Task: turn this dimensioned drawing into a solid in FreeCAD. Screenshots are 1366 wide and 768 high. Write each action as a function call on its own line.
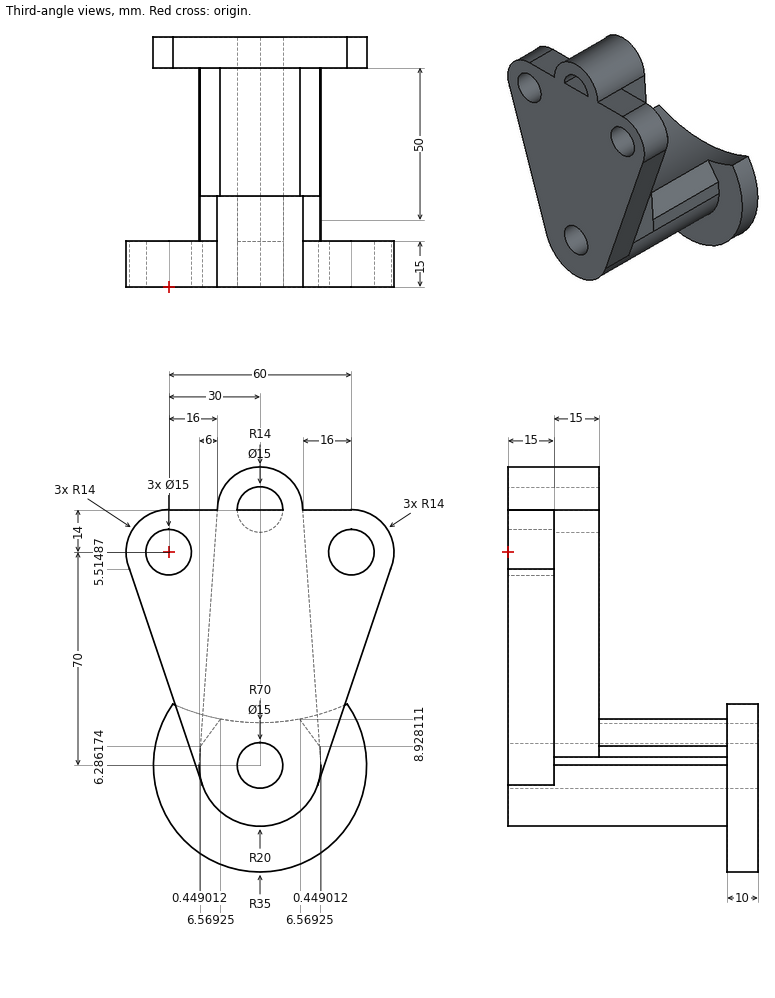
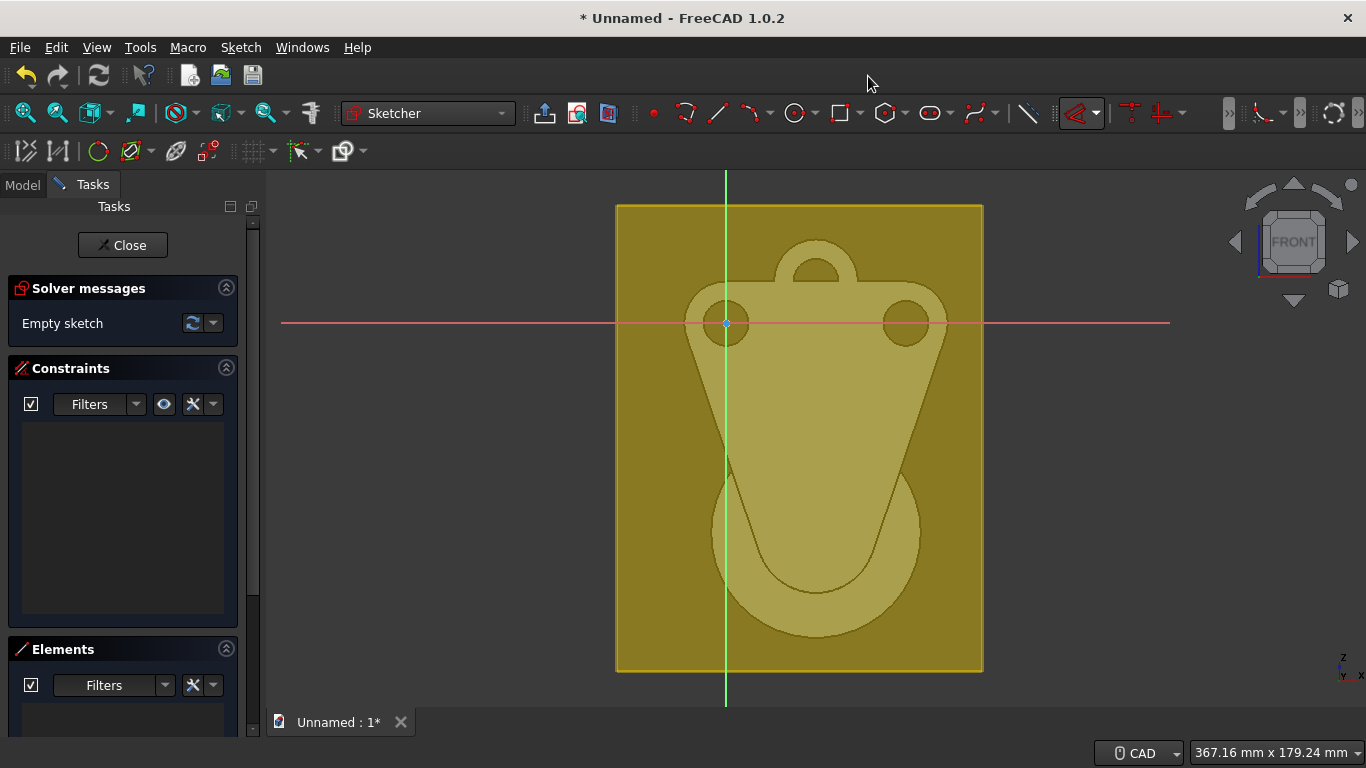
scroll(827, 548, up, 10)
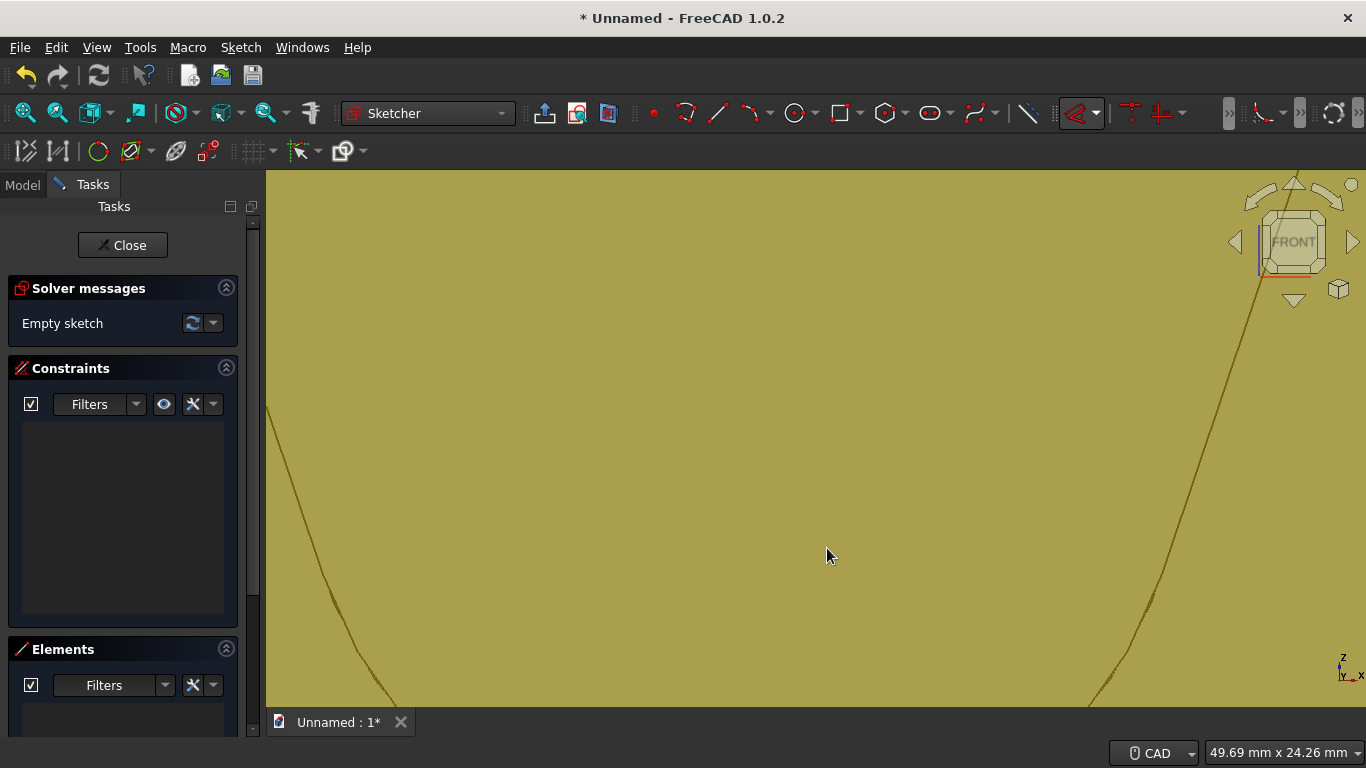
click(796, 114)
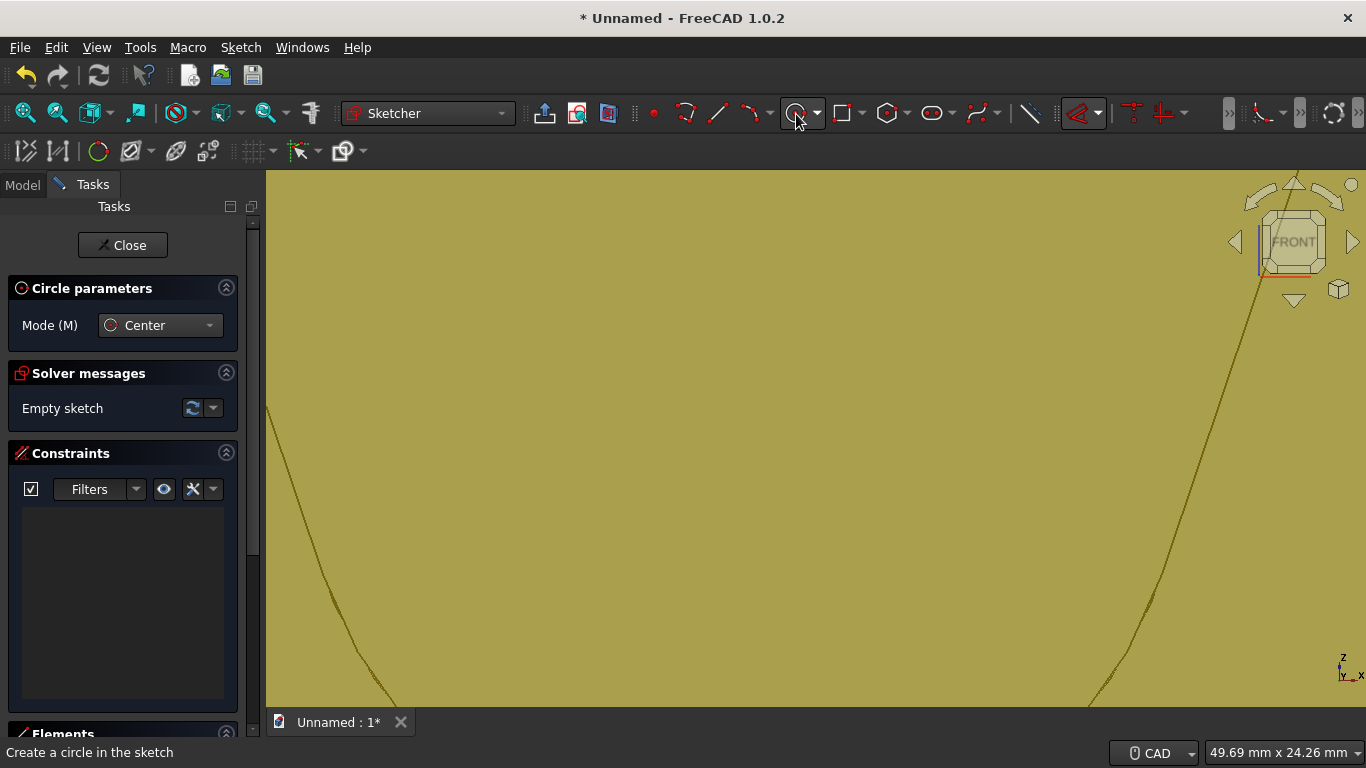
click(742, 433)
move(860, 315)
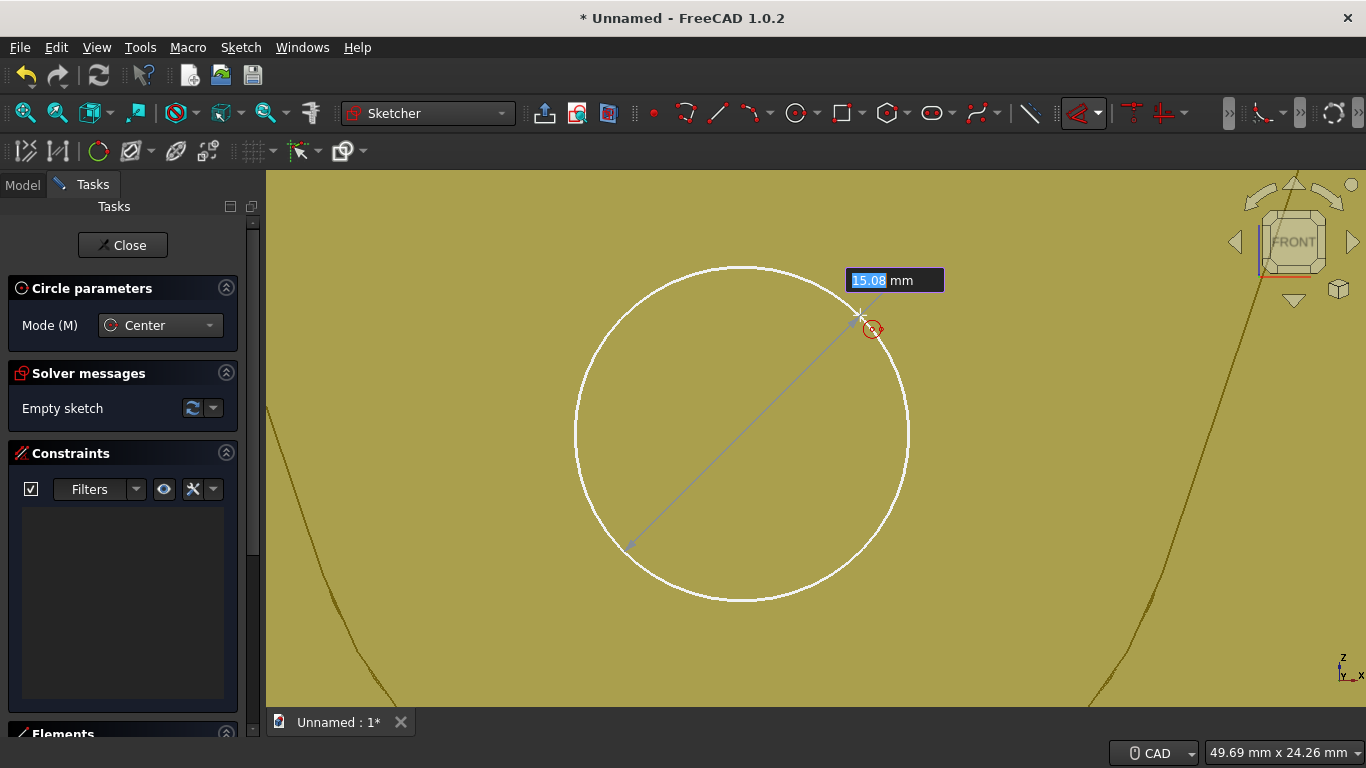
text(15)
key(Return)
key(Escape)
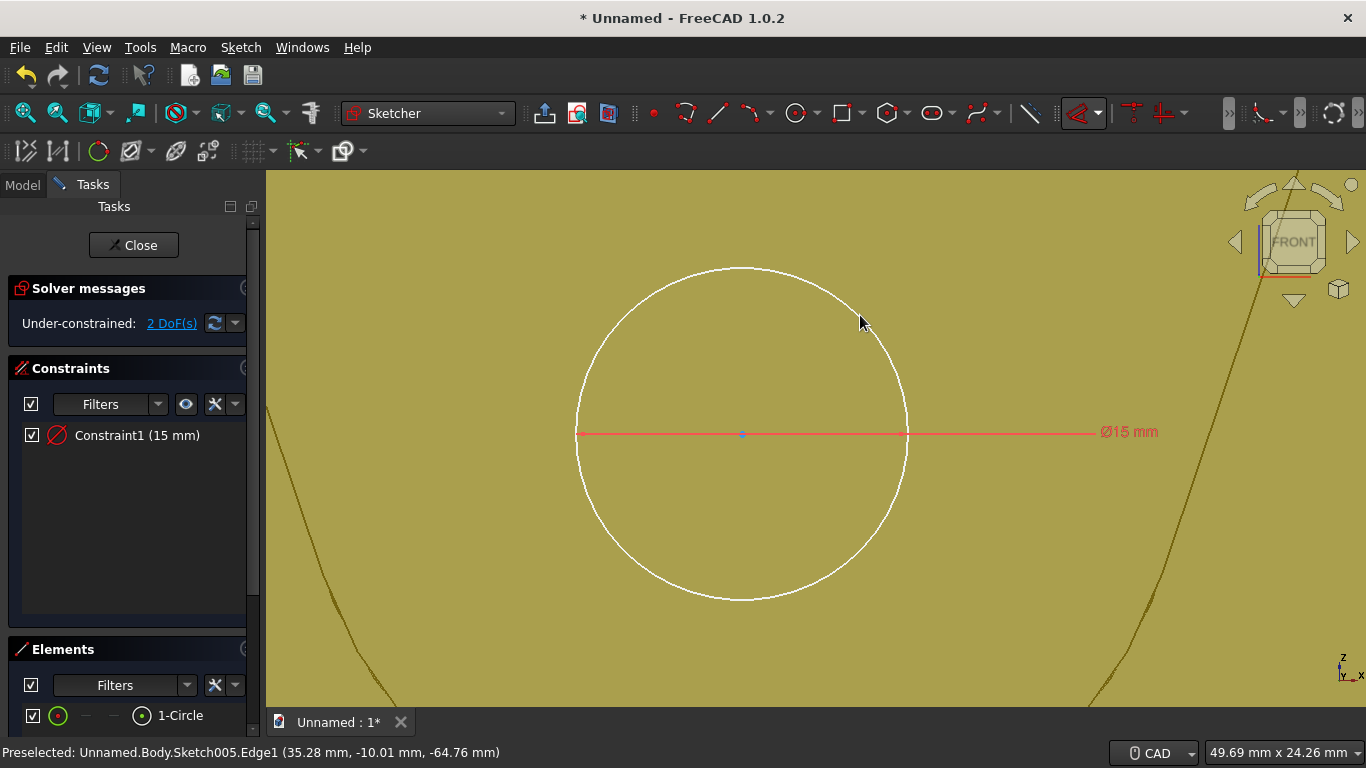
click(742, 434)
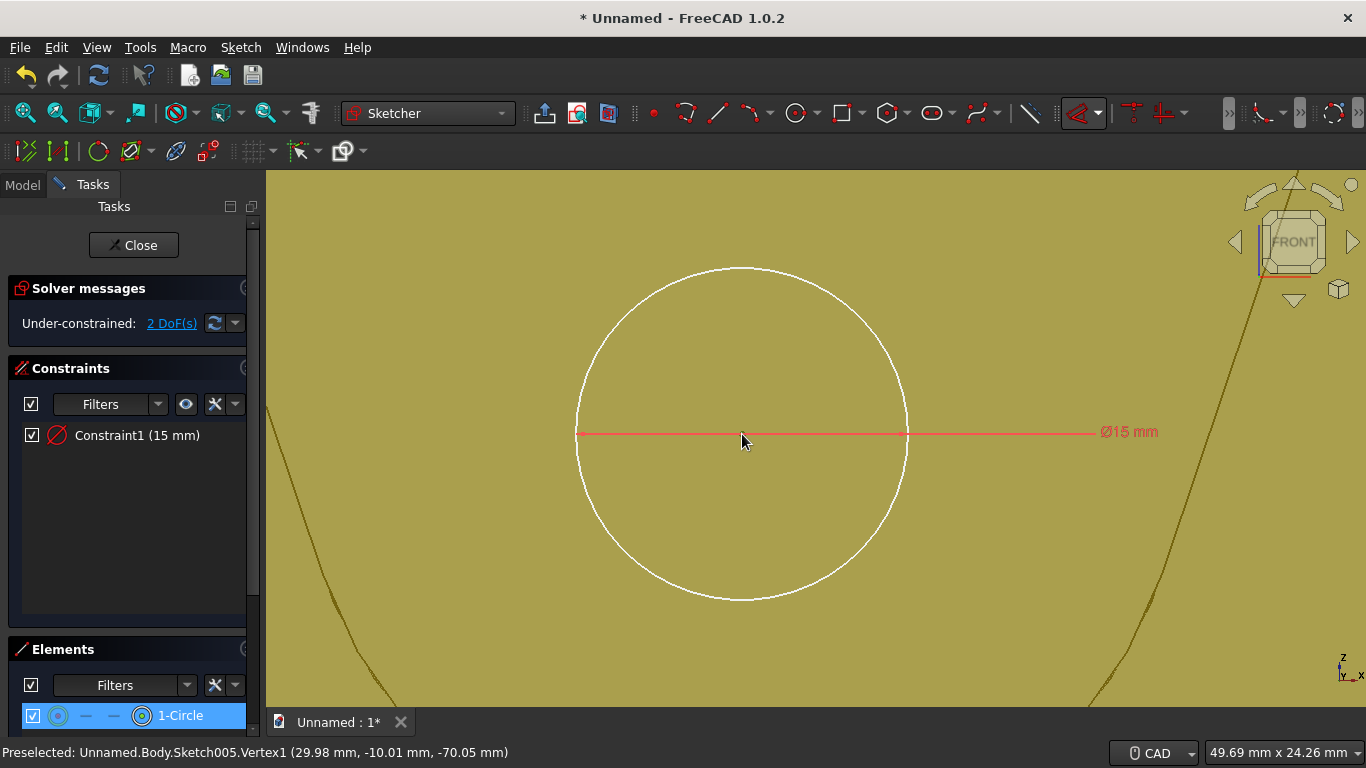
key(l)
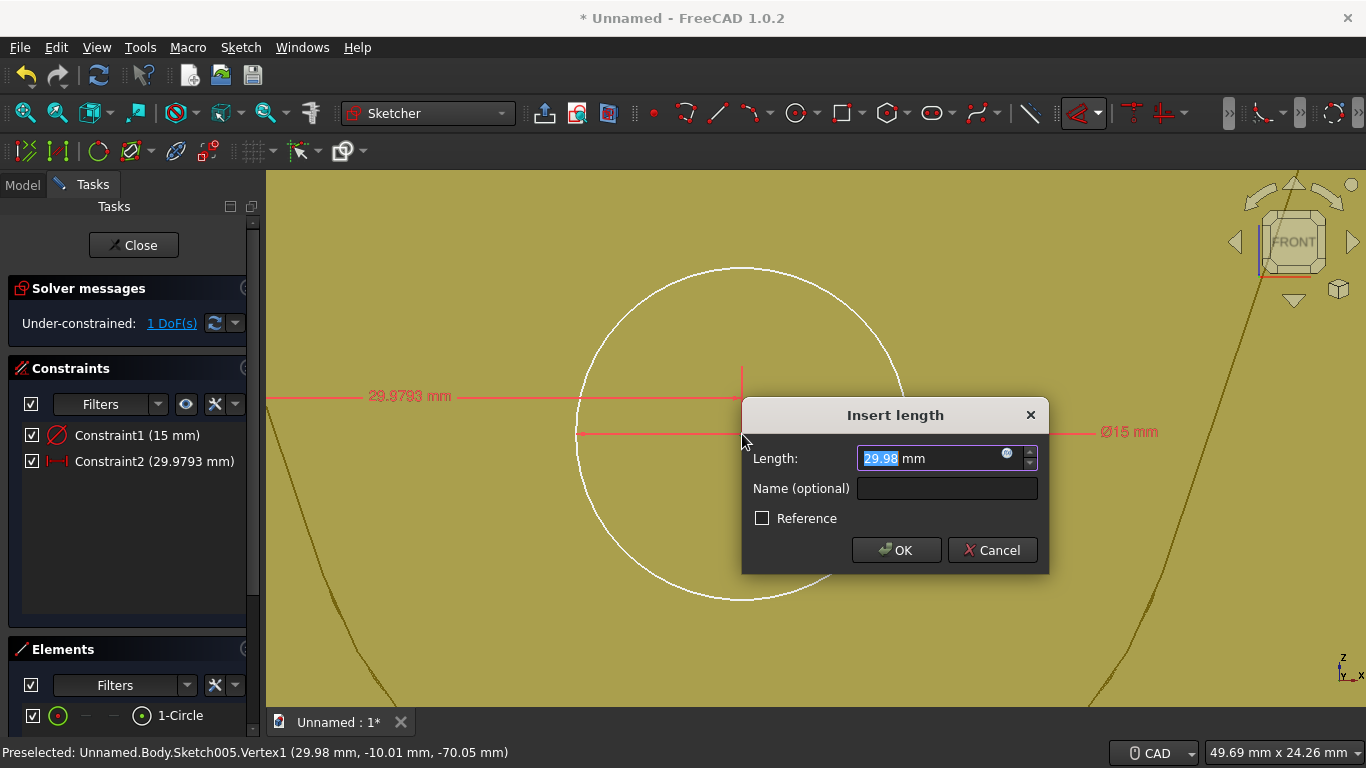
text(30)
key(Return)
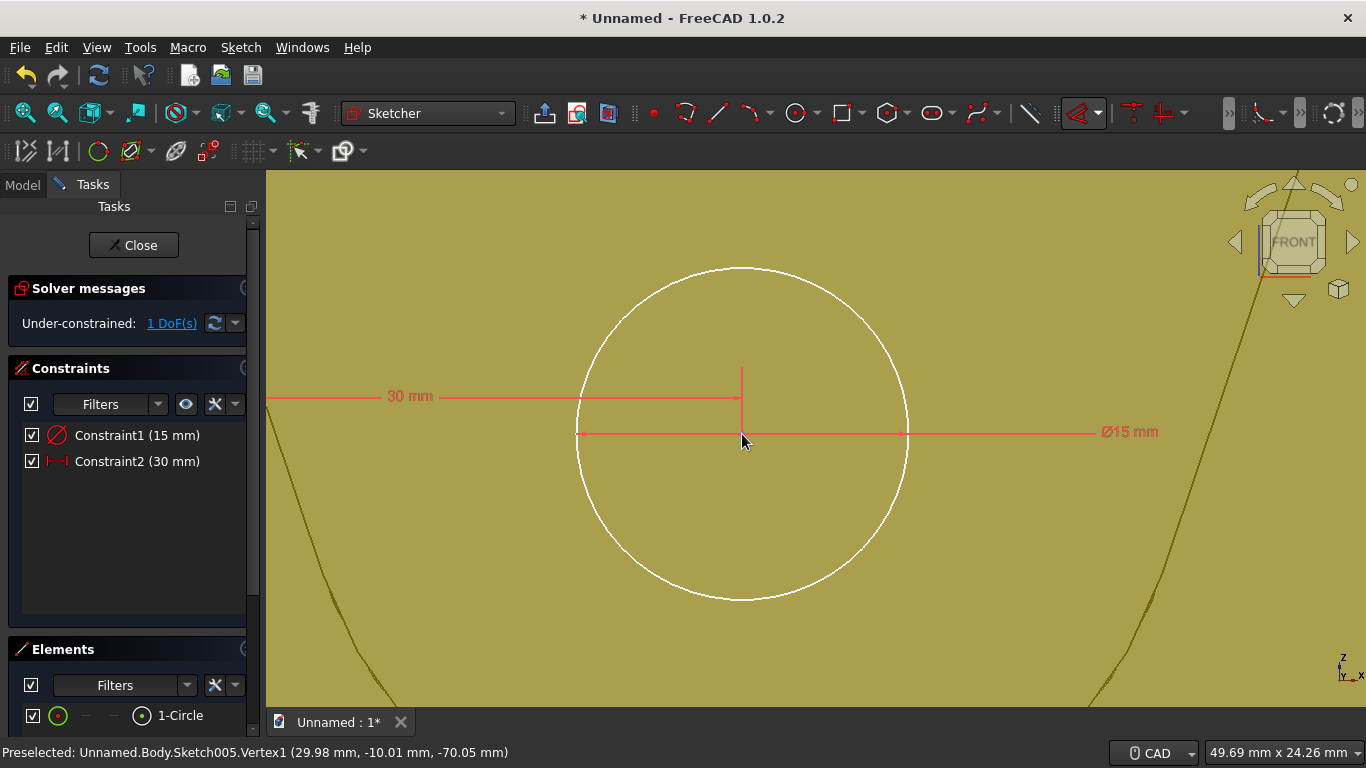
click(742, 434)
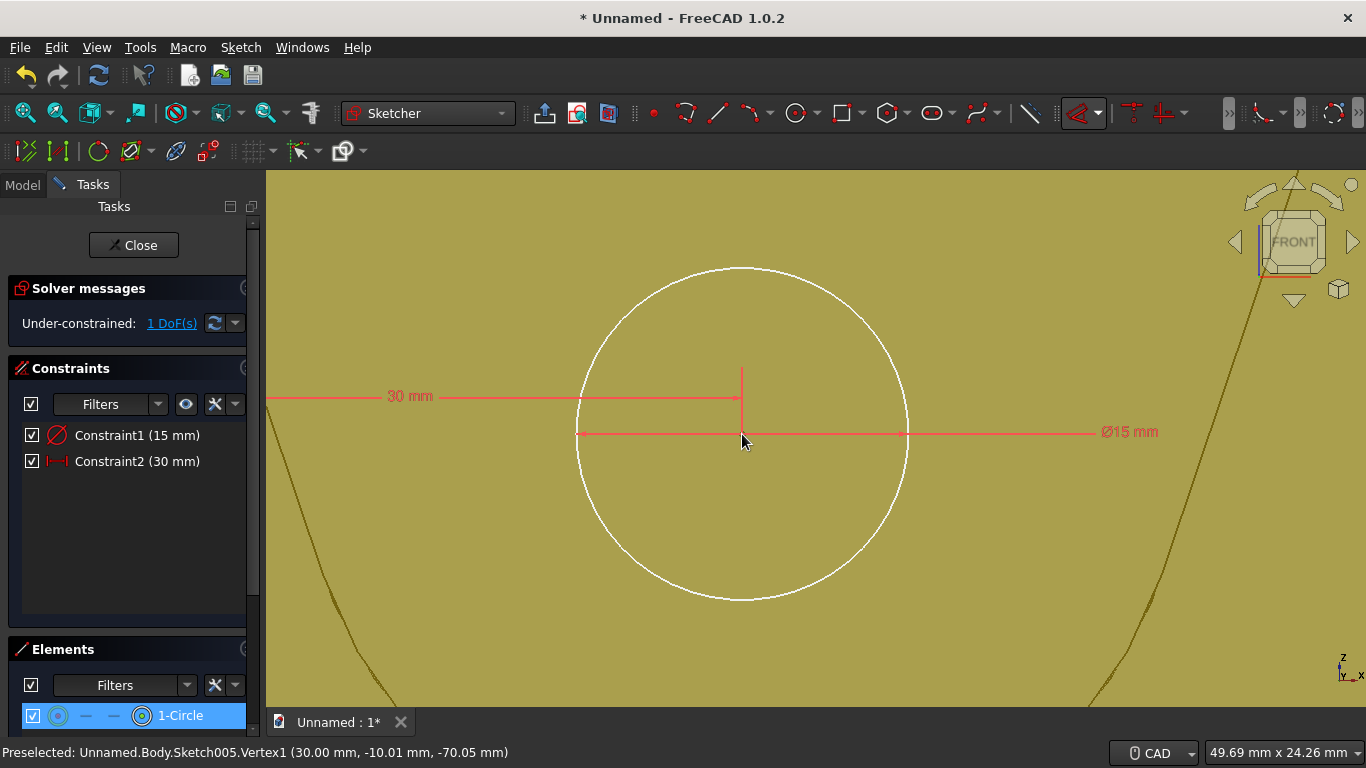
key(i)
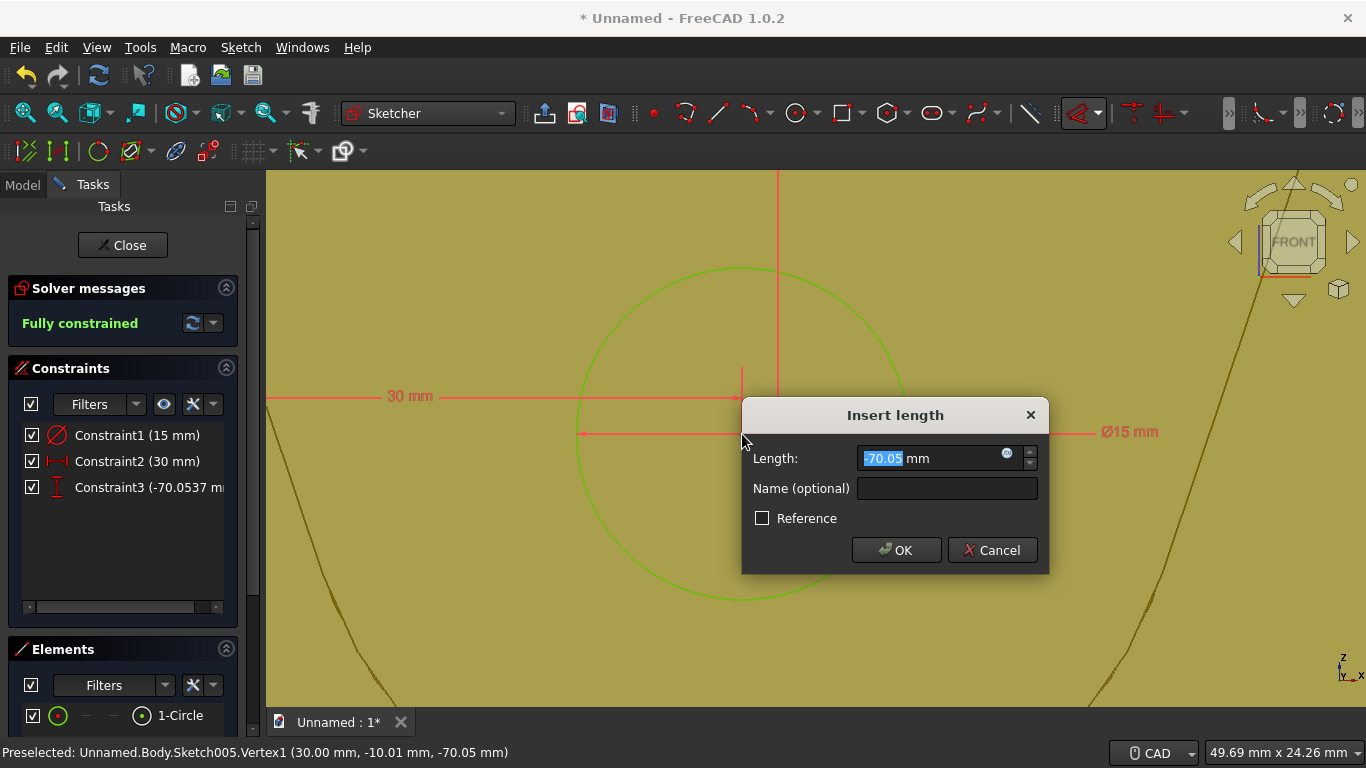
text(-70)
key(Return)